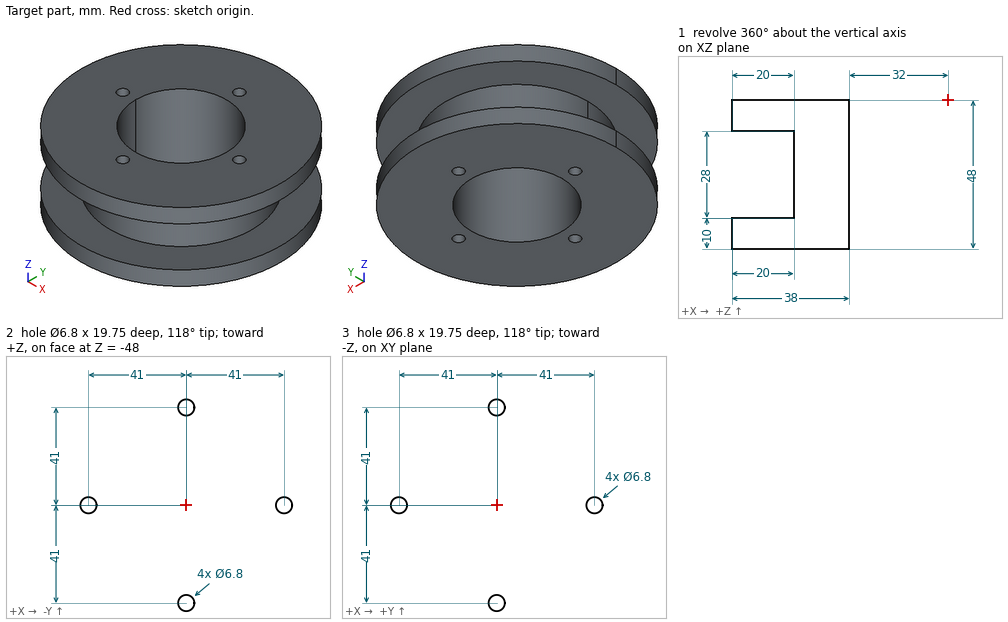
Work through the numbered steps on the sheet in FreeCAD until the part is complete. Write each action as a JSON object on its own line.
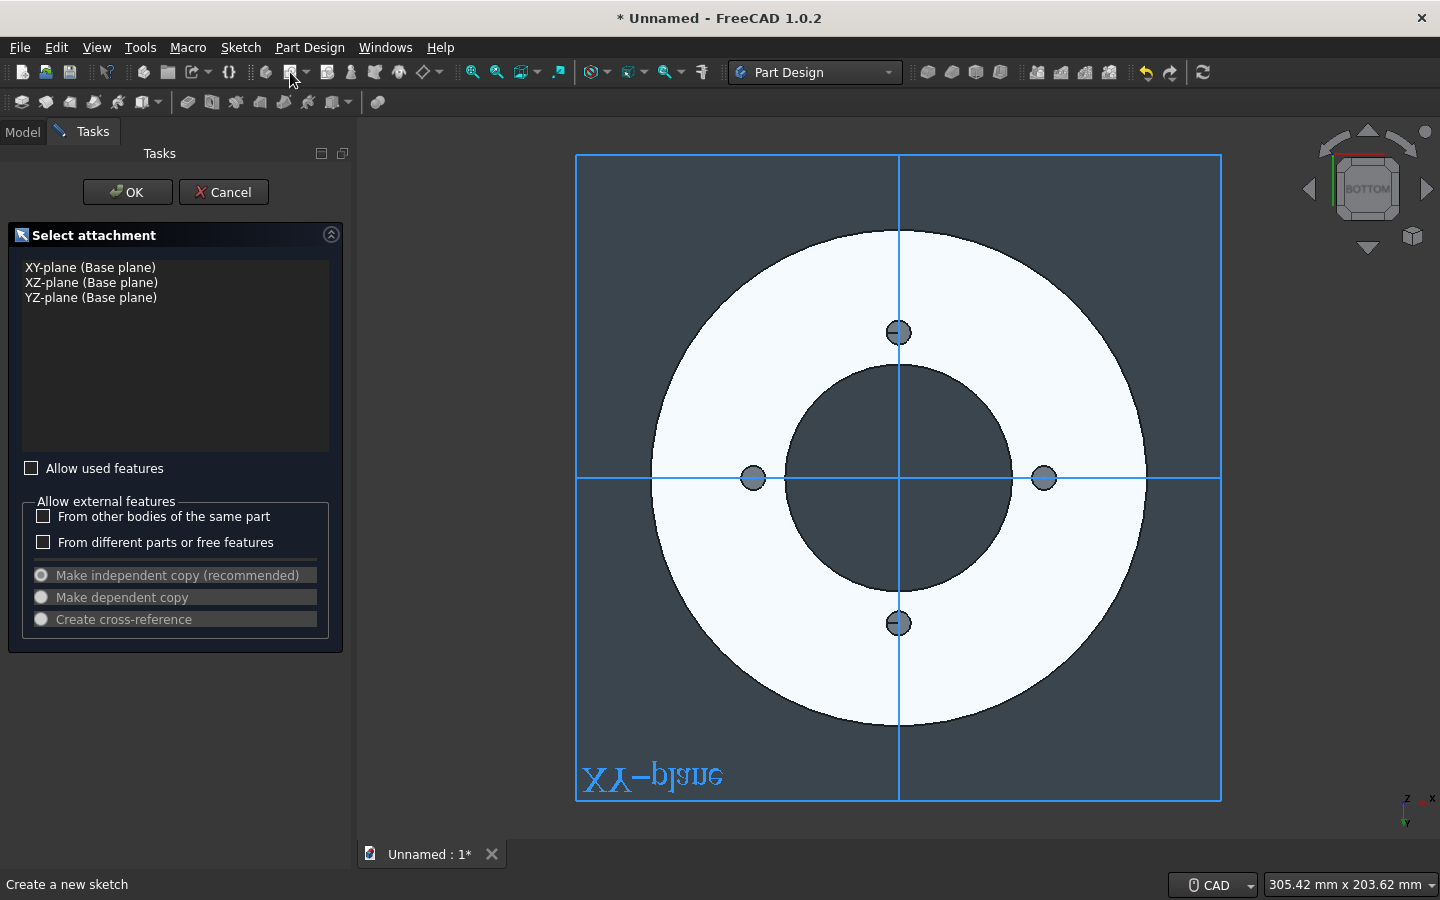
{"action": "left_click", "coordinate": [82, 268]}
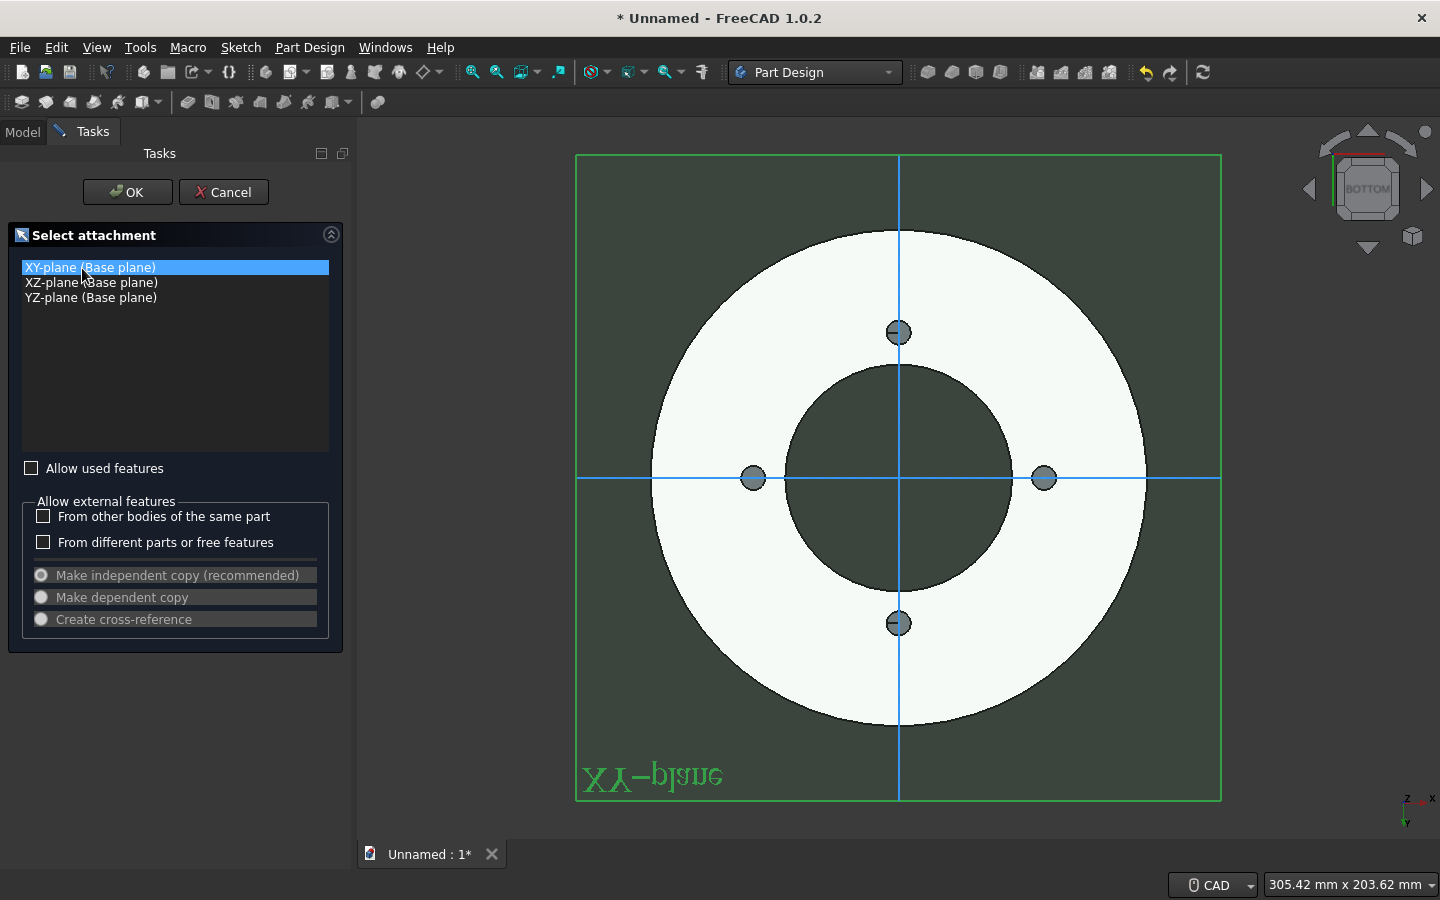
{"action": "left_click", "coordinate": [128, 192]}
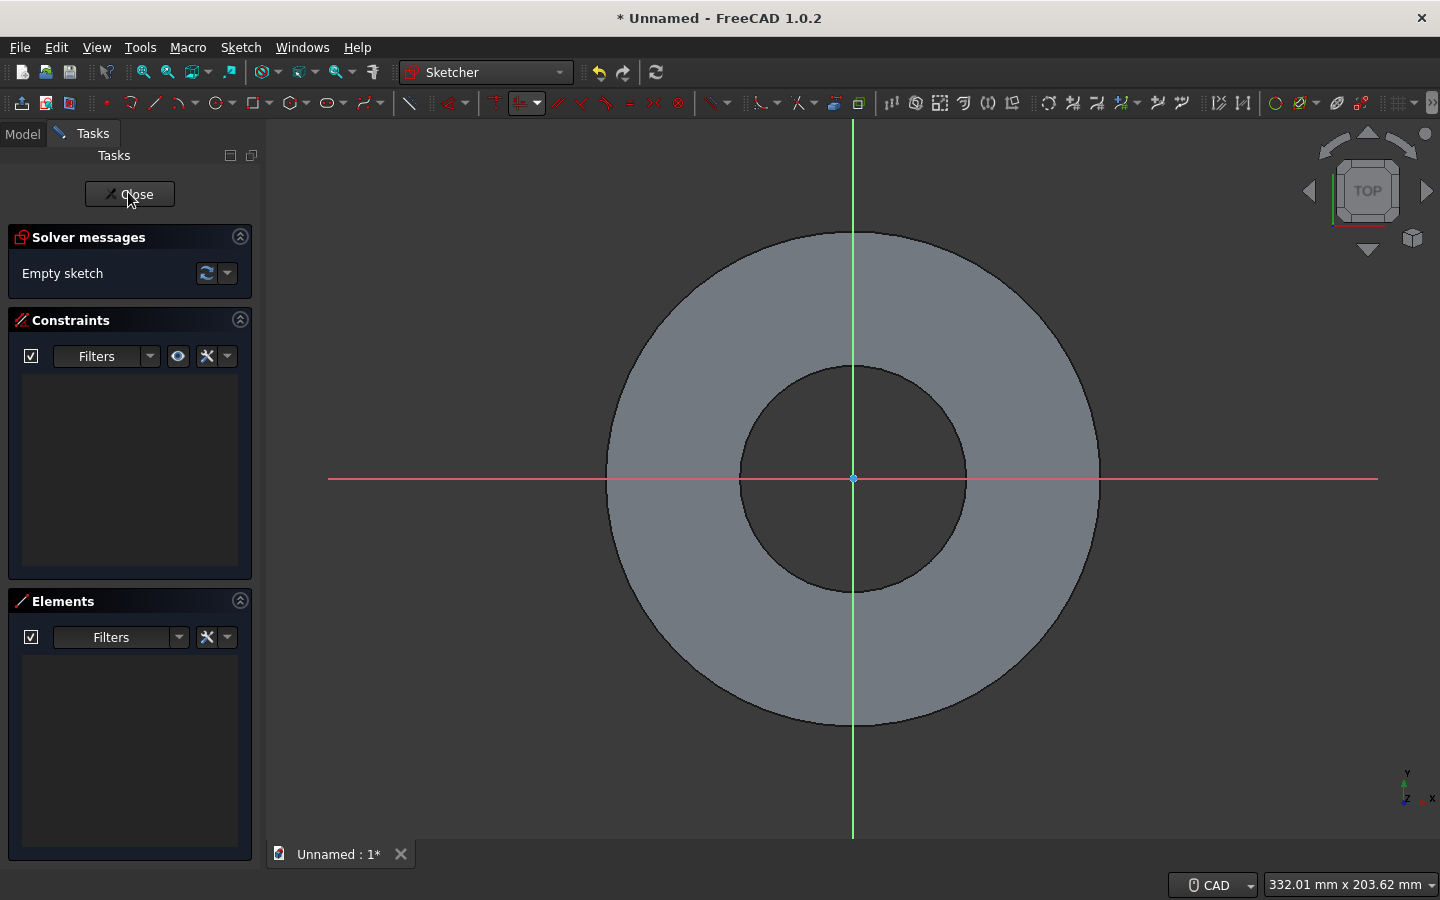
{"action": "scroll", "coordinate": [993, 479], "scroll_direction": "up", "scroll_amount": 2}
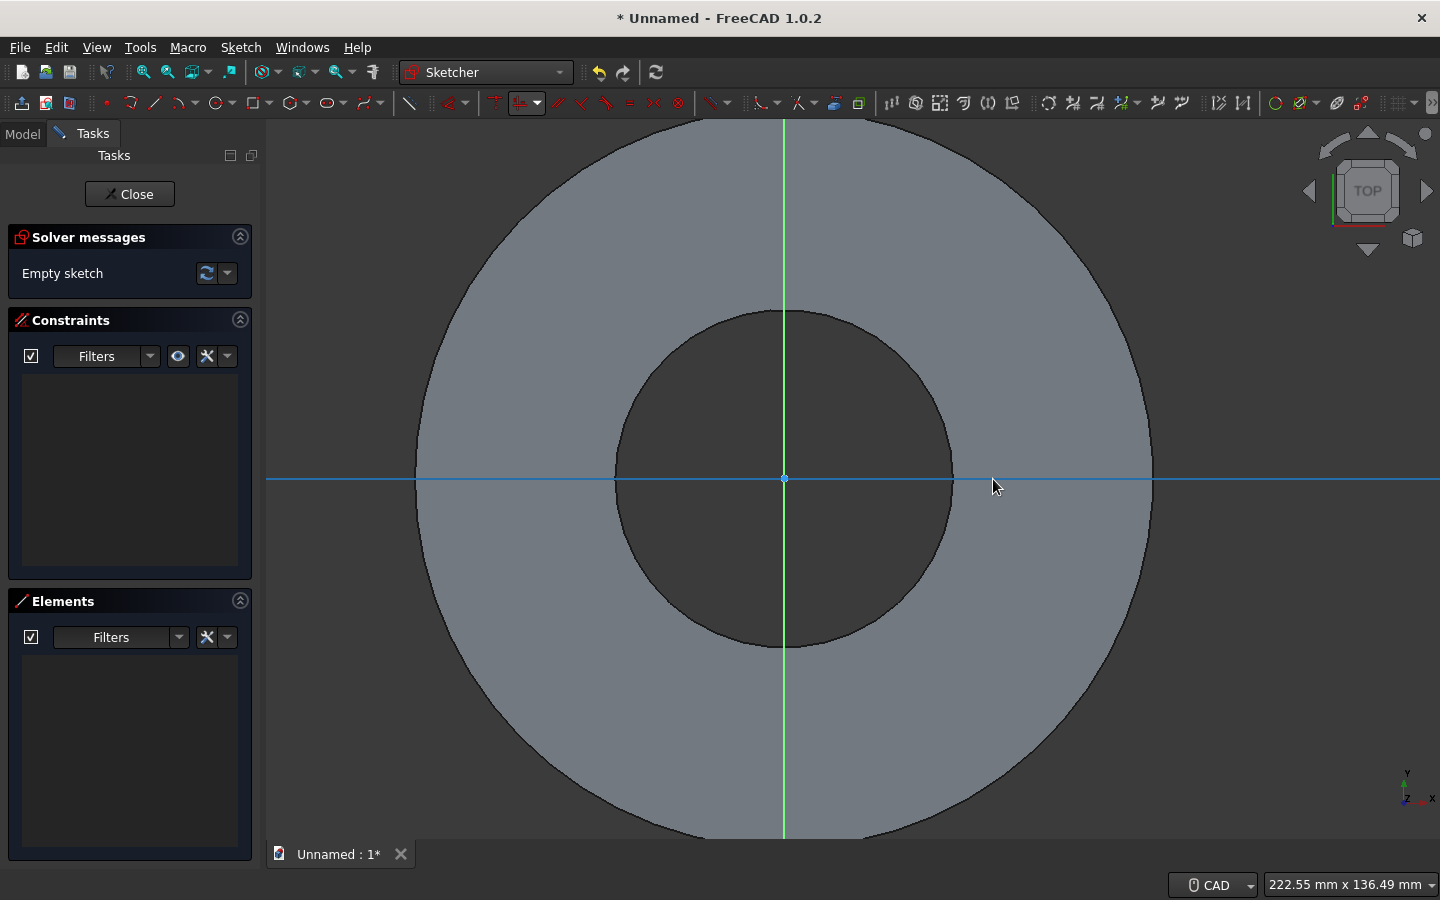
{"action": "left_click", "coordinate": [216, 104]}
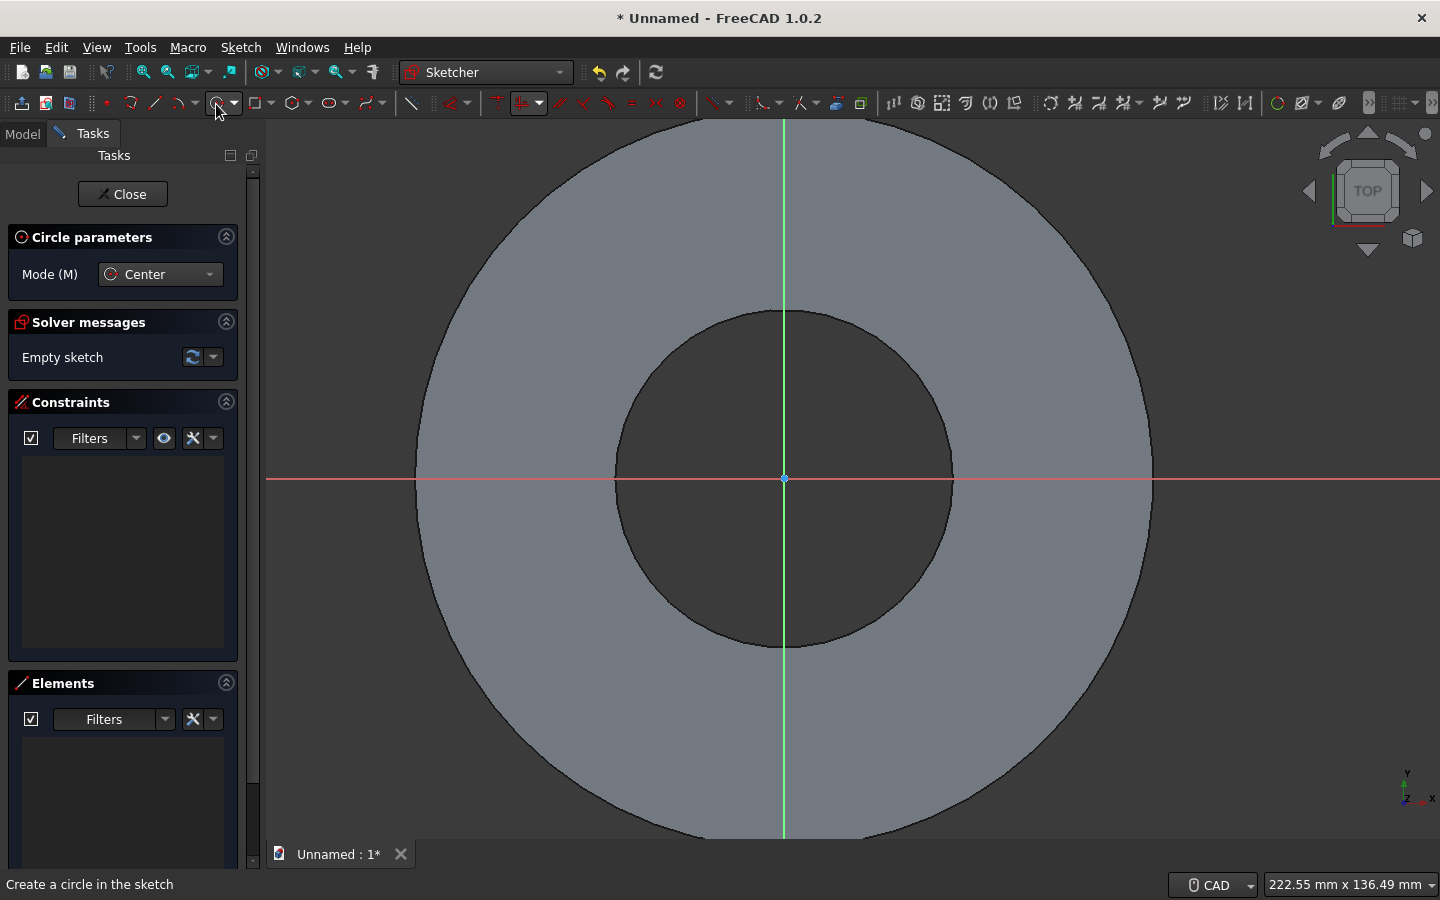
{"action": "scroll", "coordinate": [1000, 479], "scroll_direction": "up", "scroll_amount": 2}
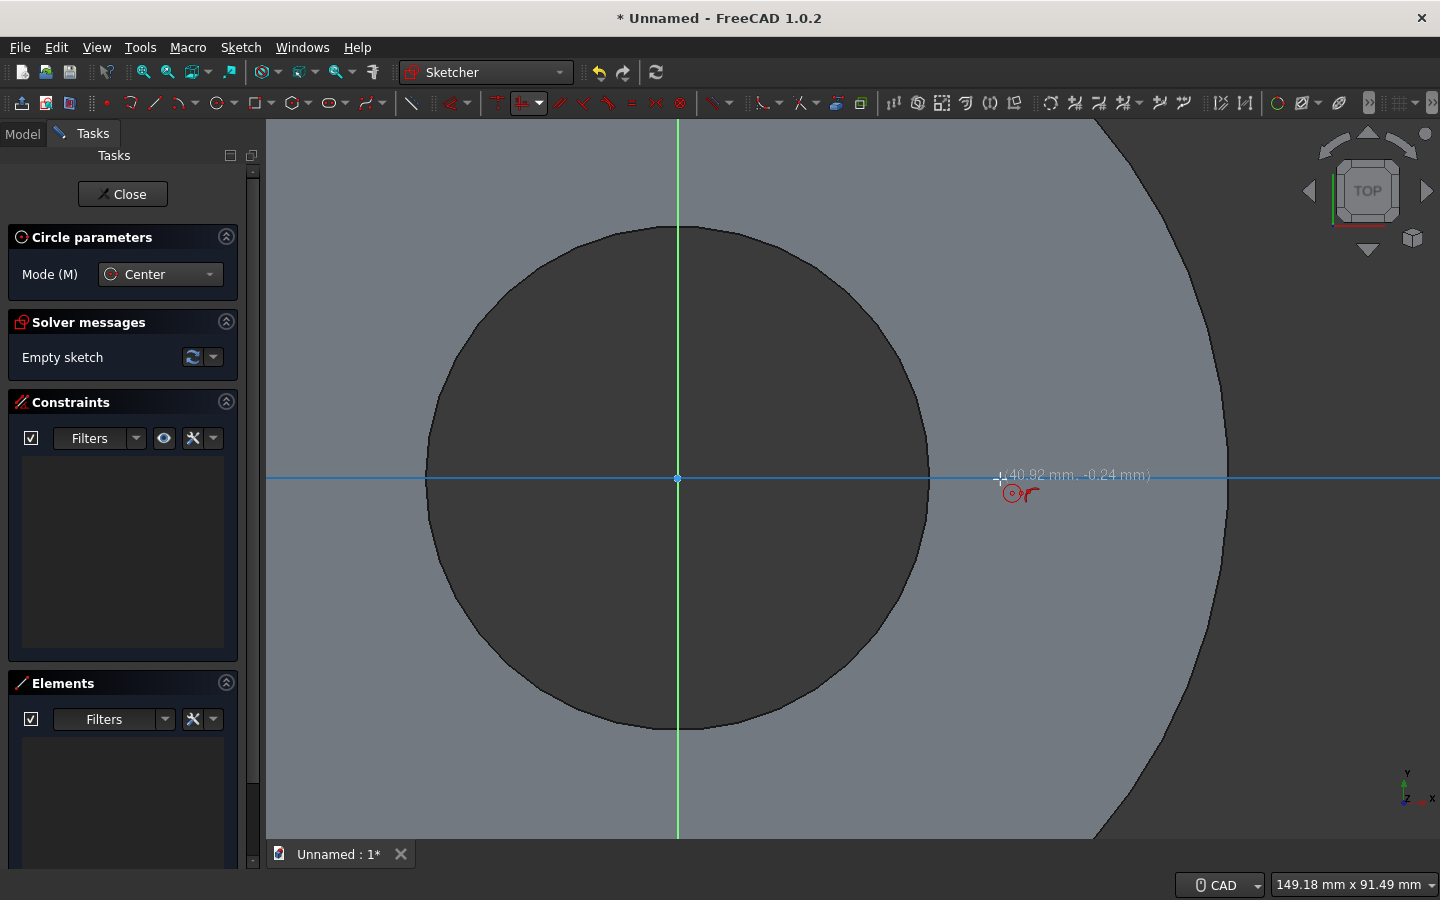
{"action": "left_click", "coordinate": [1000, 478]}
{"action": "left_click", "coordinate": [1019, 459]}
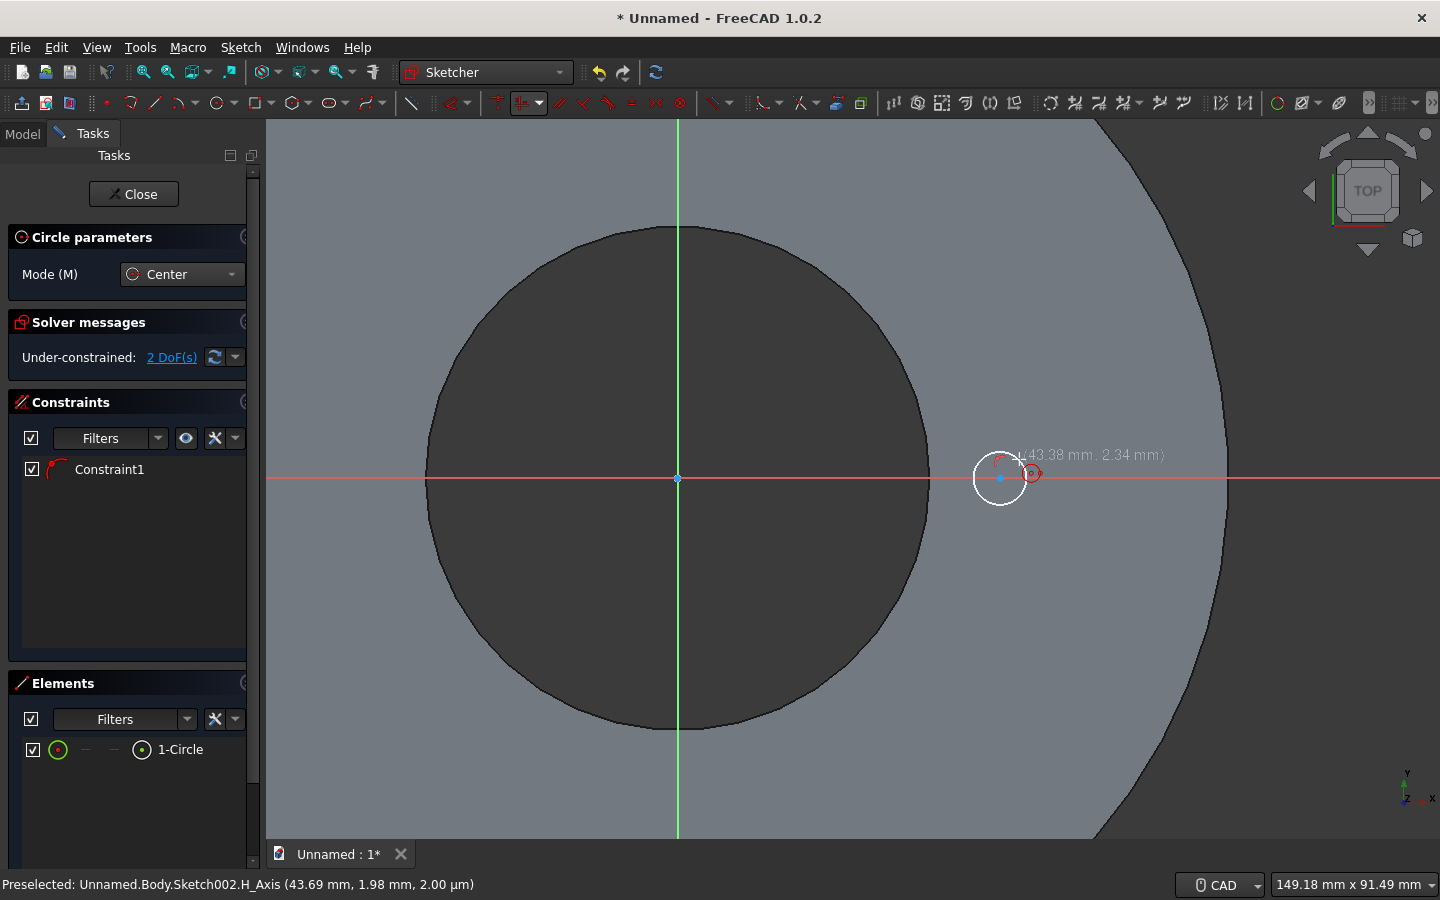
{"action": "left_click", "coordinate": [678, 801]}
{"action": "left_click", "coordinate": [697, 782]}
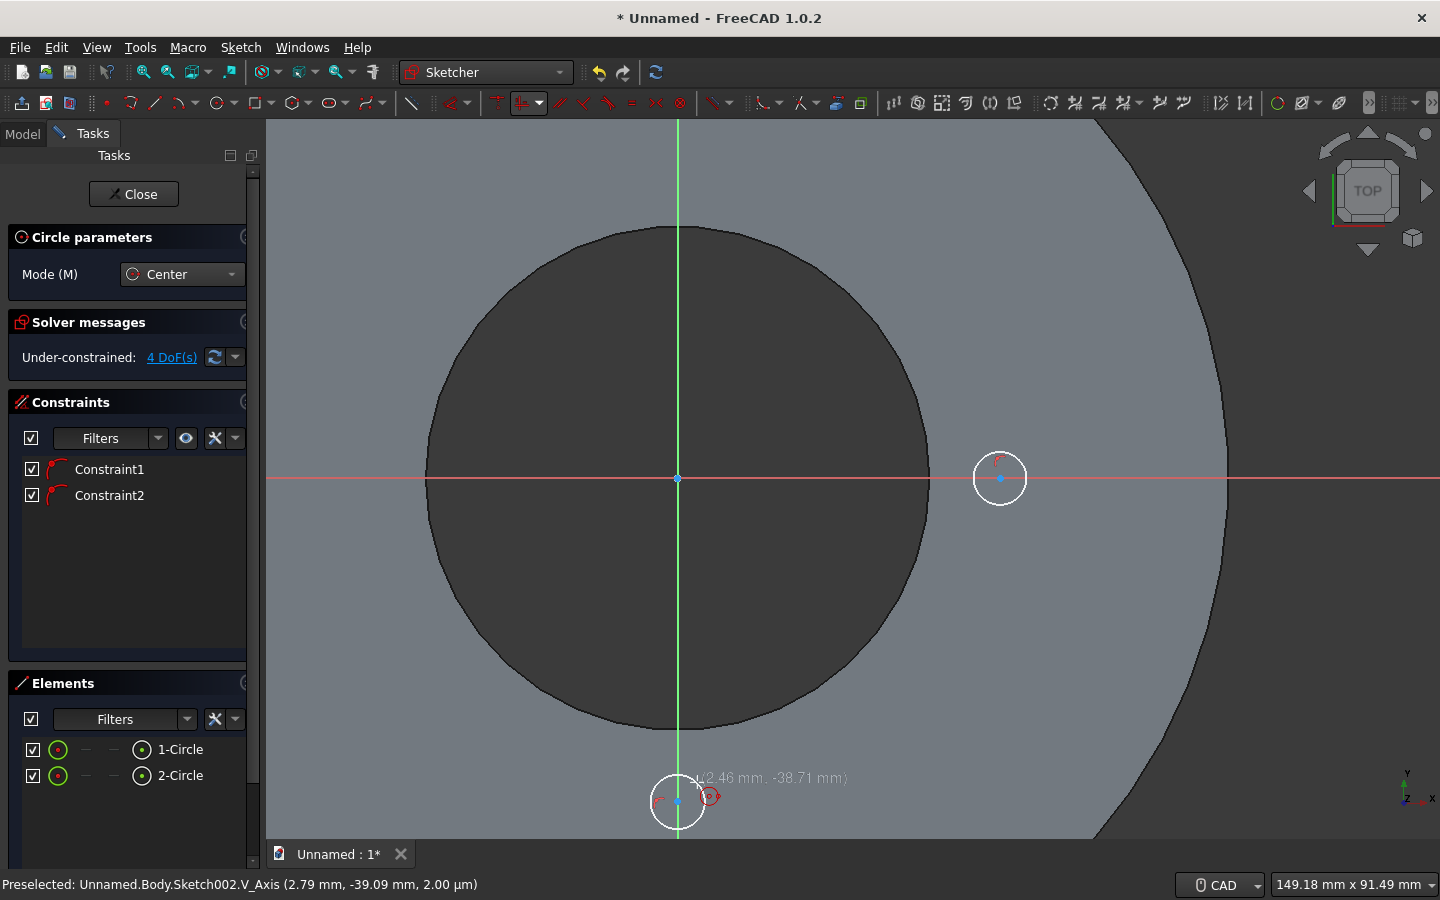
{"action": "left_click", "coordinate": [355, 478]}
{"action": "left_click", "coordinate": [374, 459]}